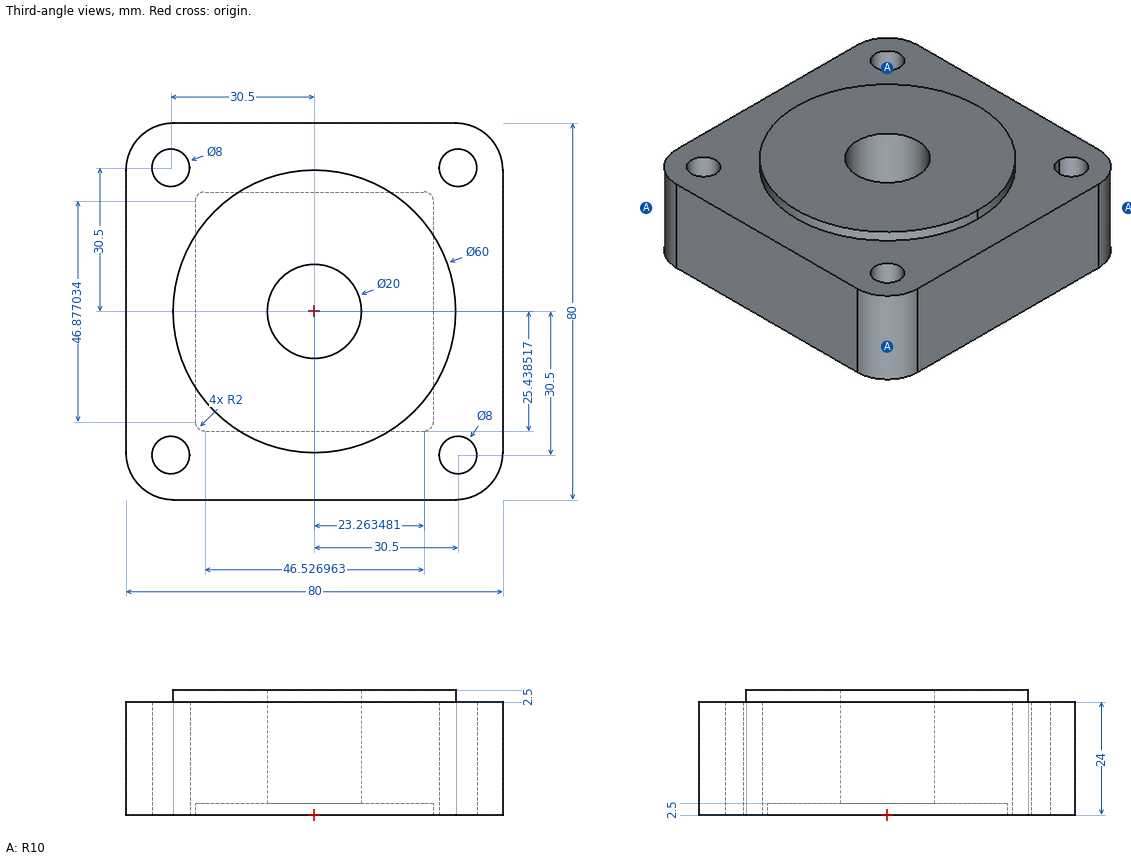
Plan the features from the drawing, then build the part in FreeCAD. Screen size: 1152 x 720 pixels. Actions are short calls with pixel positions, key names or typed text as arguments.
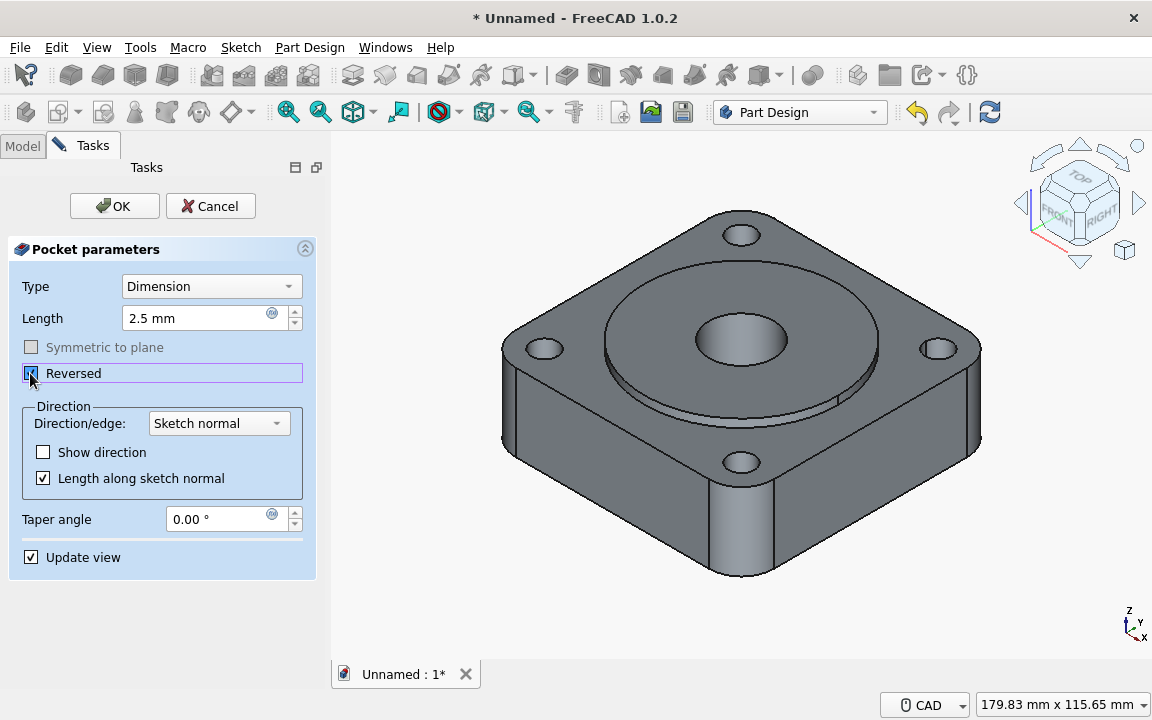
click(115, 206)